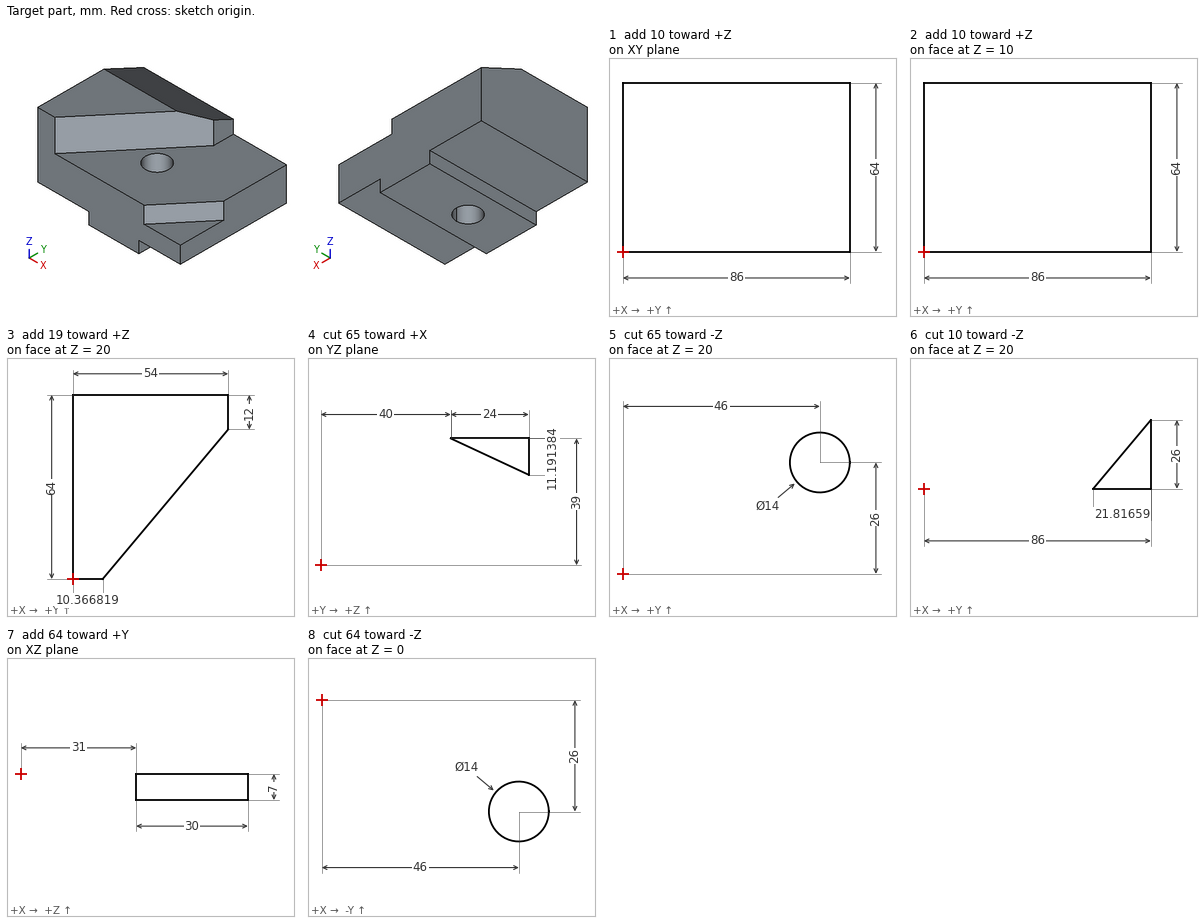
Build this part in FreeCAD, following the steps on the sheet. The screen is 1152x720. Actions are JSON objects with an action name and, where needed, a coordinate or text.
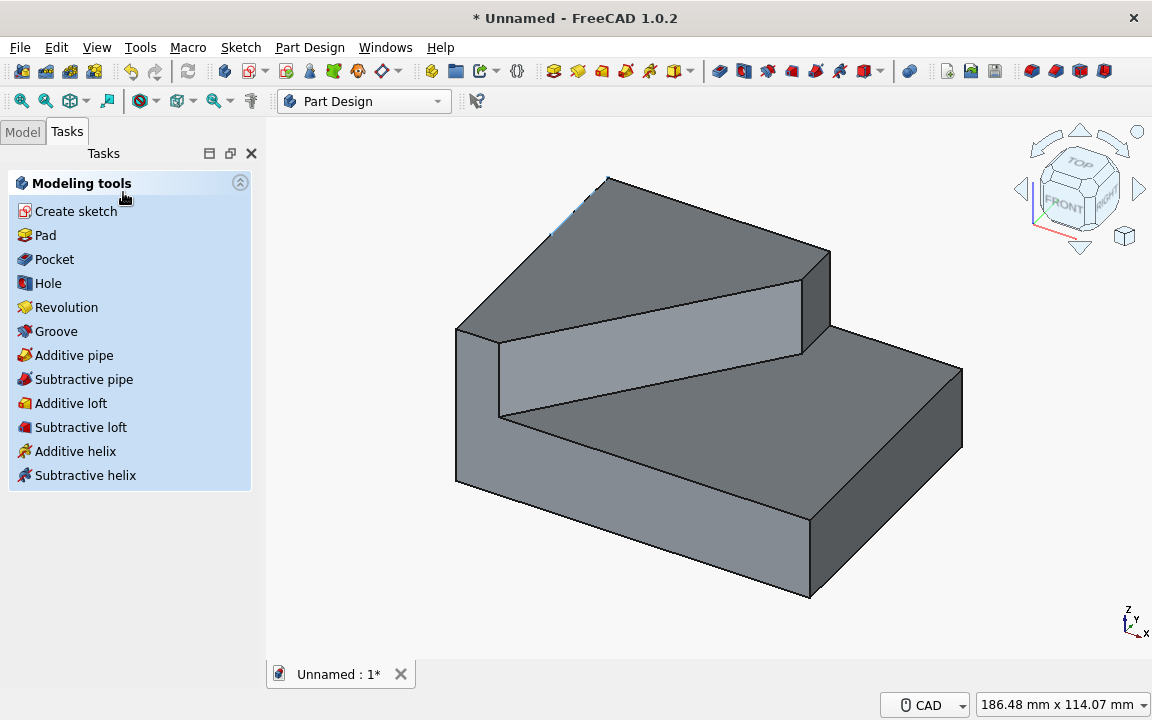
{"action": "left_click", "coordinate": [720, 72]}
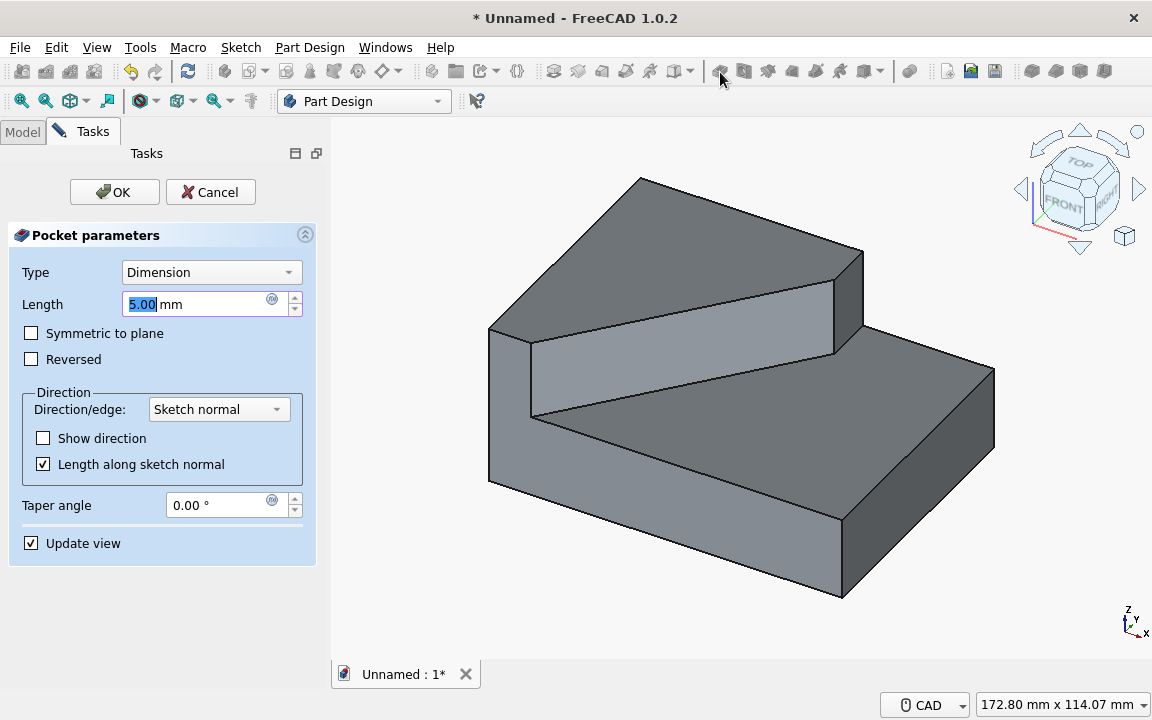
{"action": "type", "text": "65"}
{"action": "key", "text": "Tab"}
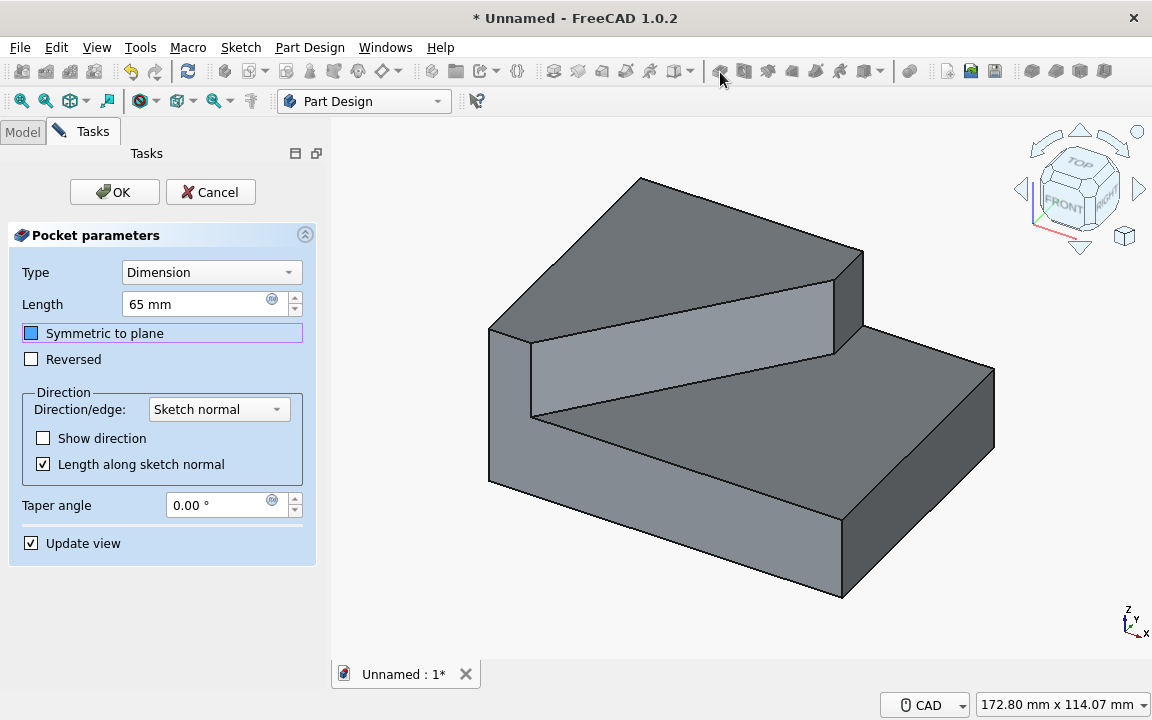
{"action": "left_click", "coordinate": [30, 359]}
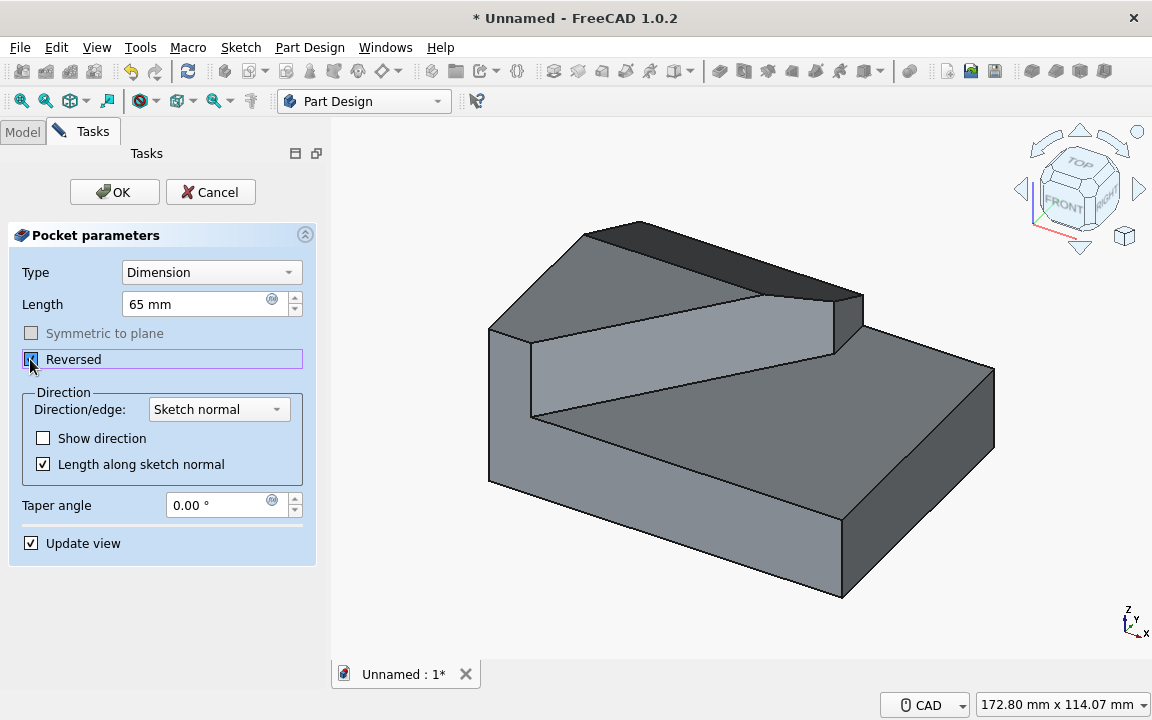
{"action": "left_click", "coordinate": [115, 192]}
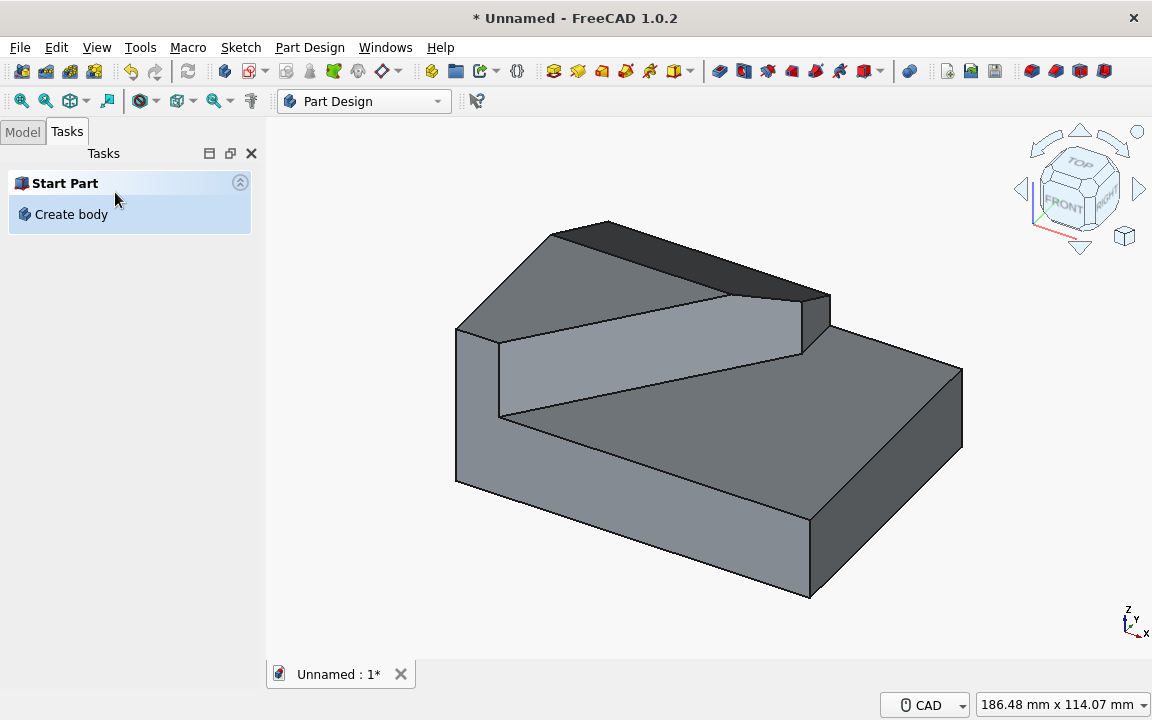
{"action": "left_click", "coordinate": [753, 428]}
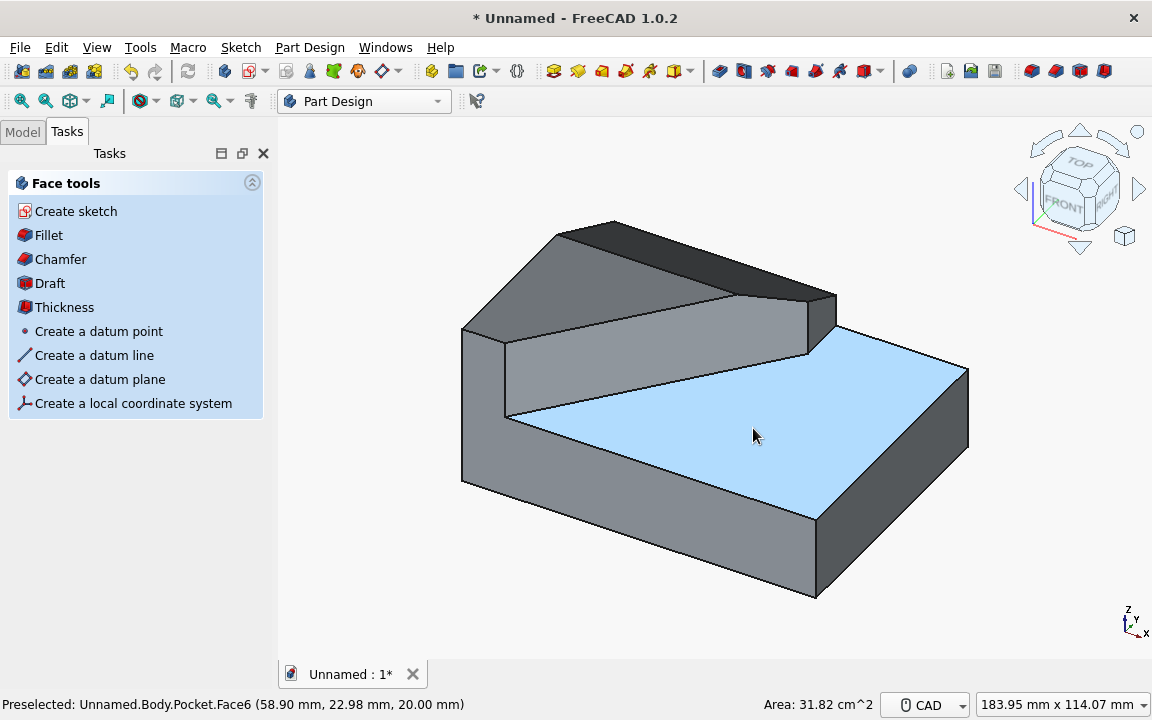
{"action": "left_click", "coordinate": [250, 72]}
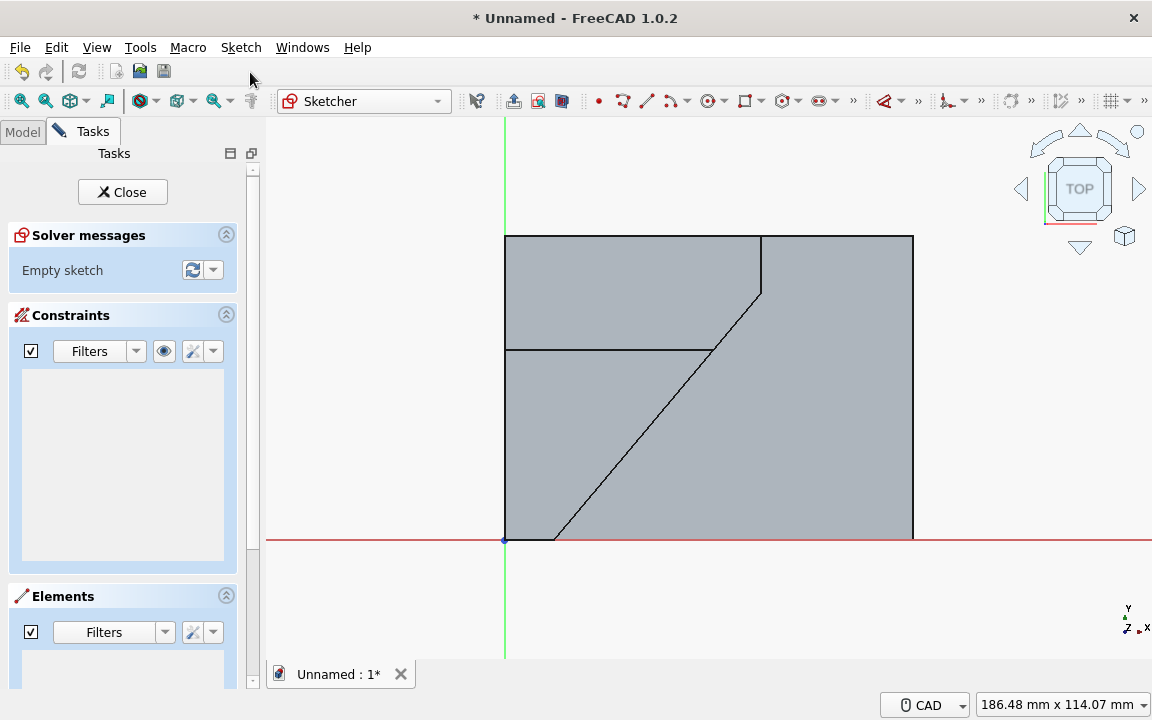
{"action": "scroll", "coordinate": [744, 424], "scroll_direction": "up", "scroll_amount": 8}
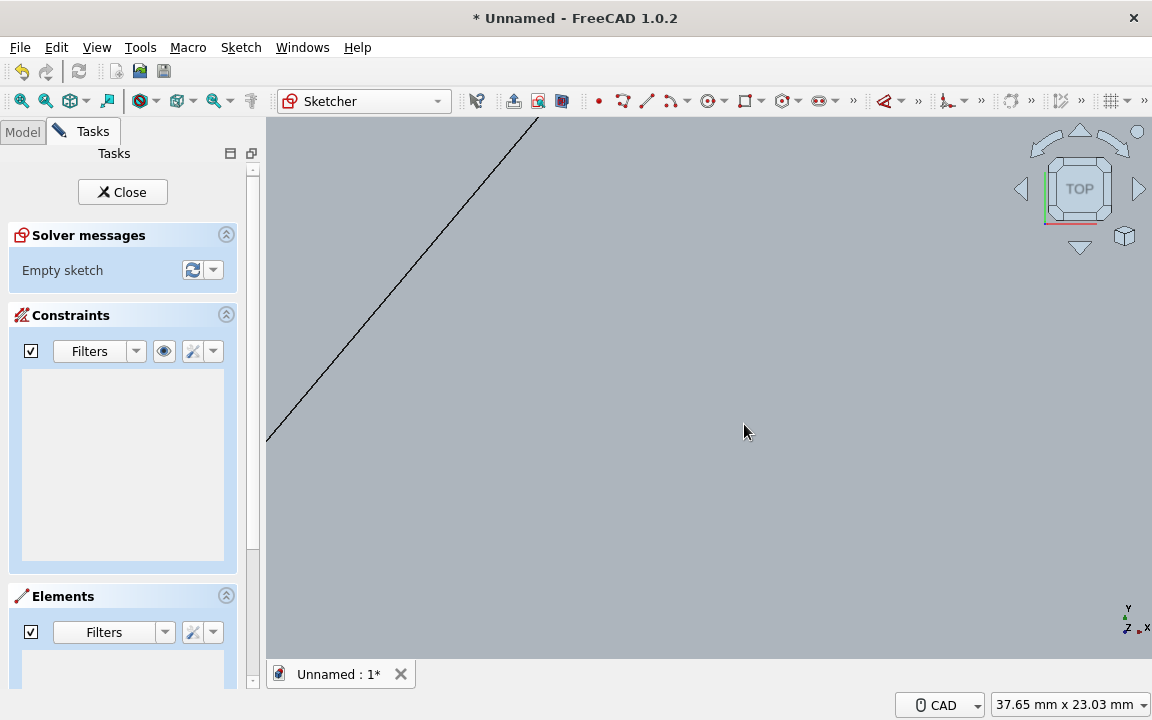
{"action": "left_click", "coordinate": [708, 102]}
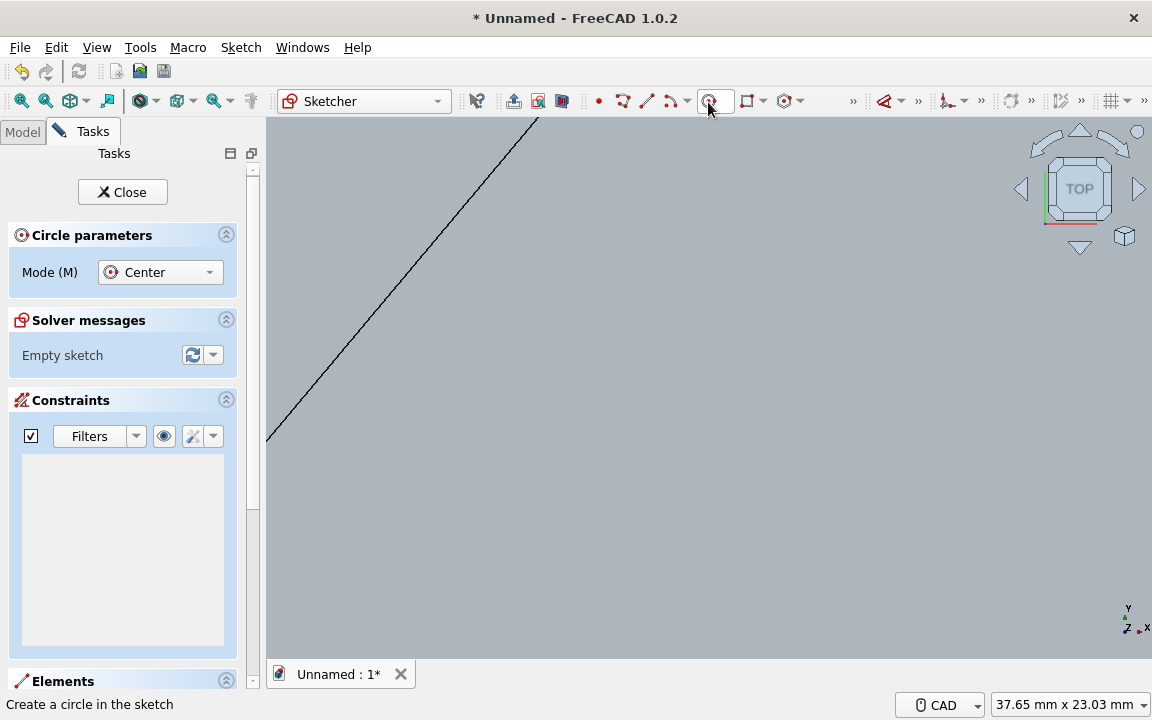
{"action": "left_click", "coordinate": [639, 385]}
{"action": "mouse_move", "coordinate": [756, 268]}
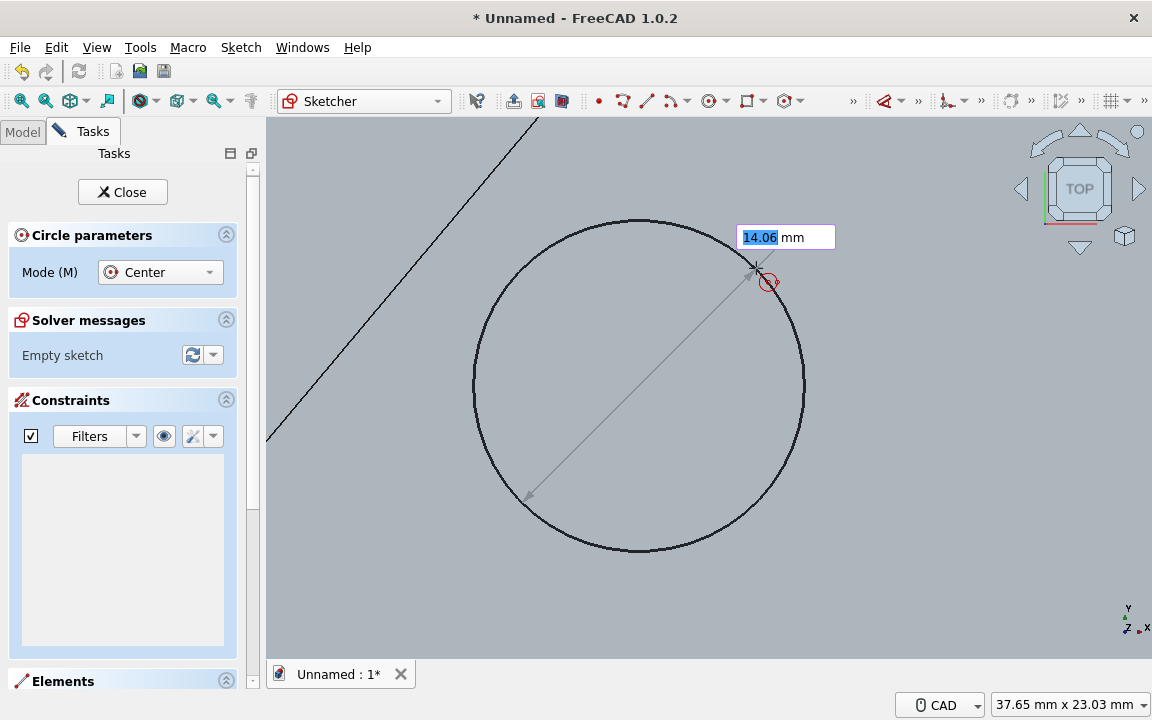
{"action": "type", "text": "14"}
{"action": "key", "text": "Return"}
{"action": "key", "text": "Escape"}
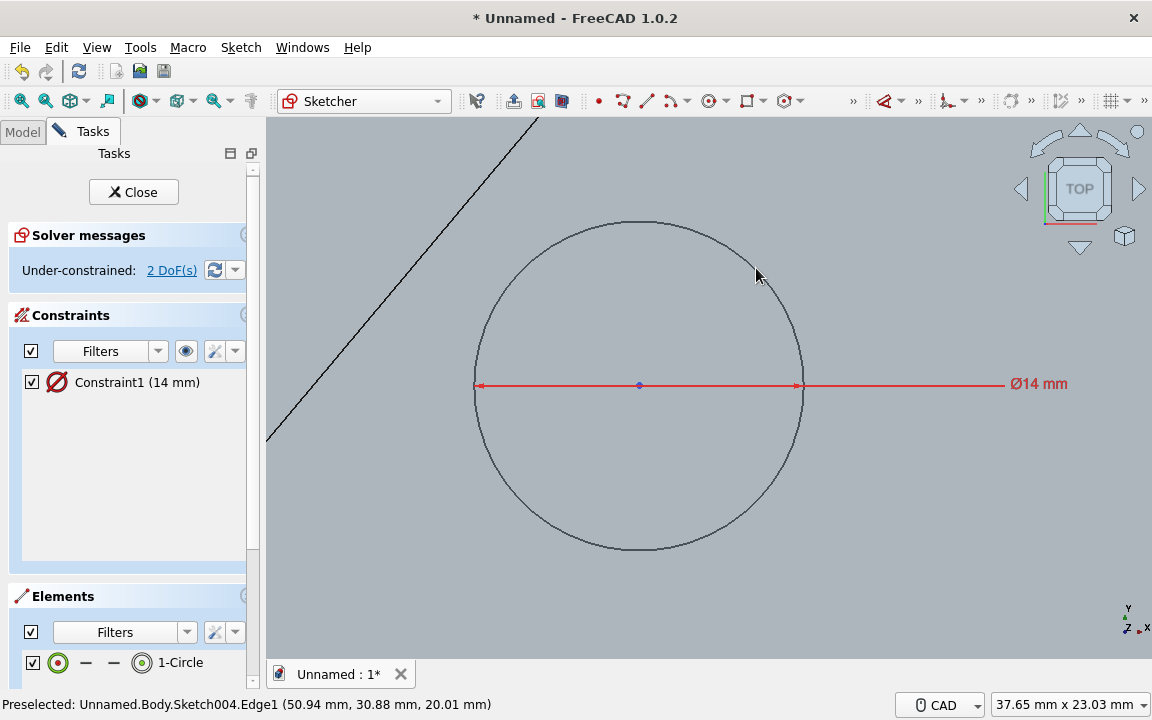
{"action": "left_click", "coordinate": [884, 102]}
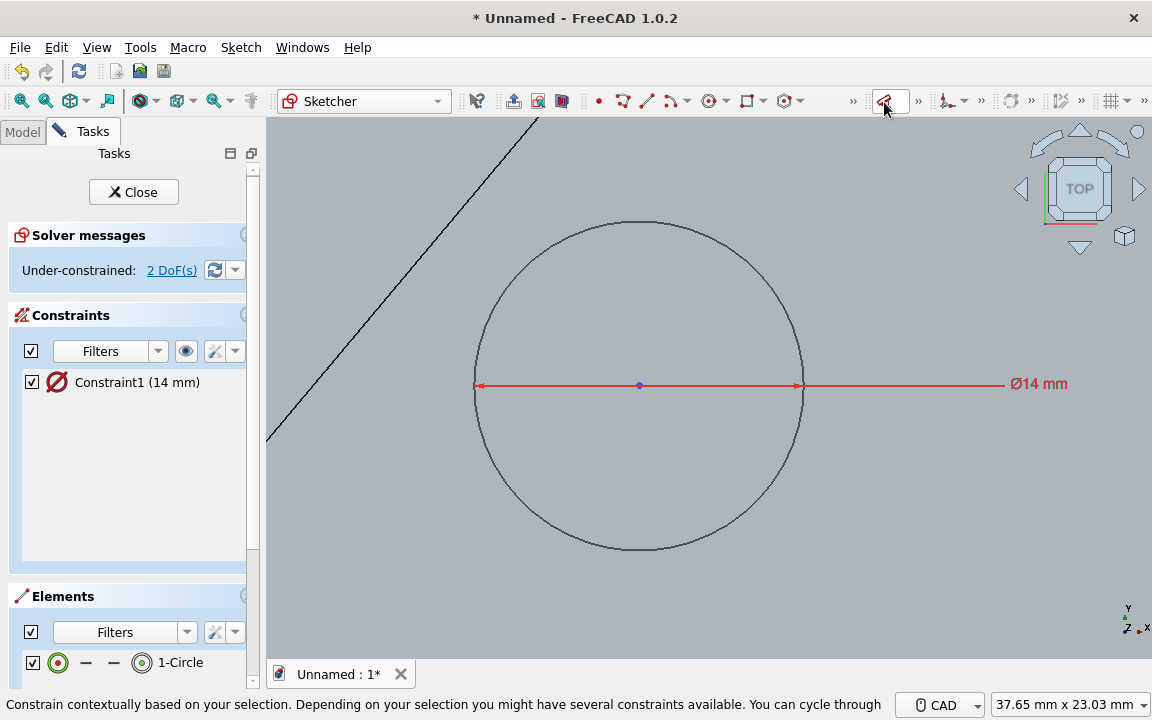
{"action": "left_click", "coordinate": [639, 386]}
{"action": "left_click", "coordinate": [387, 352]}